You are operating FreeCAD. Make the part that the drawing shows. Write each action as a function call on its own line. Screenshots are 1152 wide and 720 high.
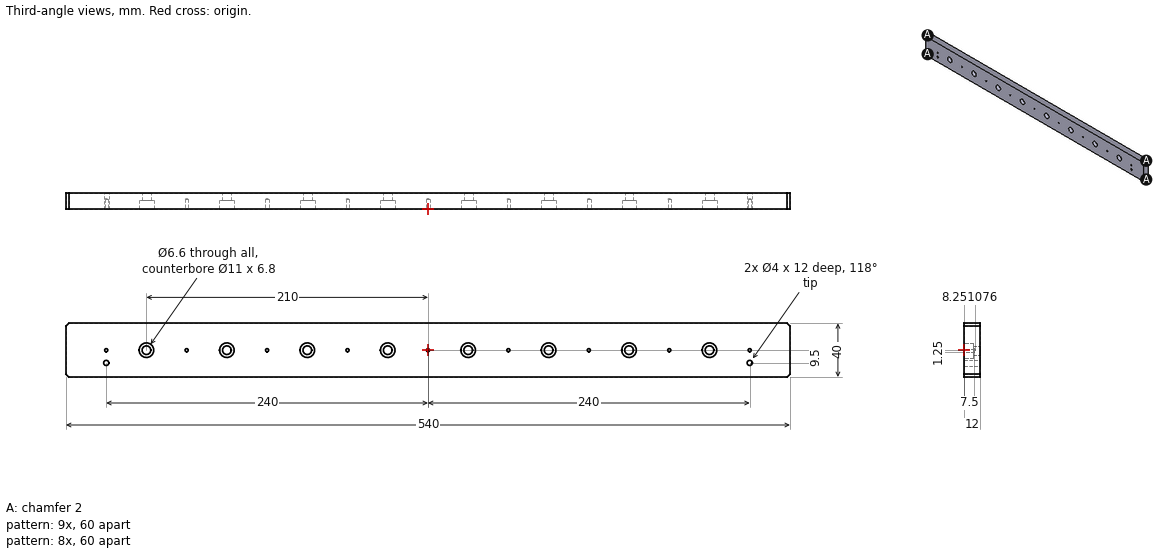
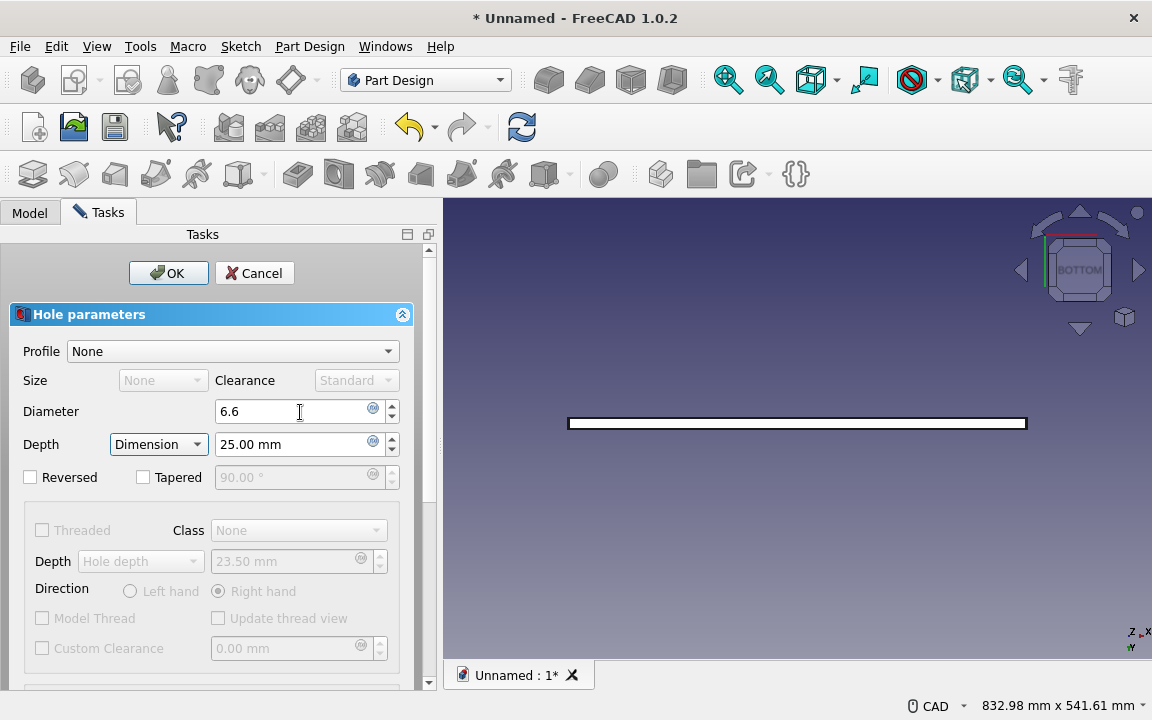
click(160, 444)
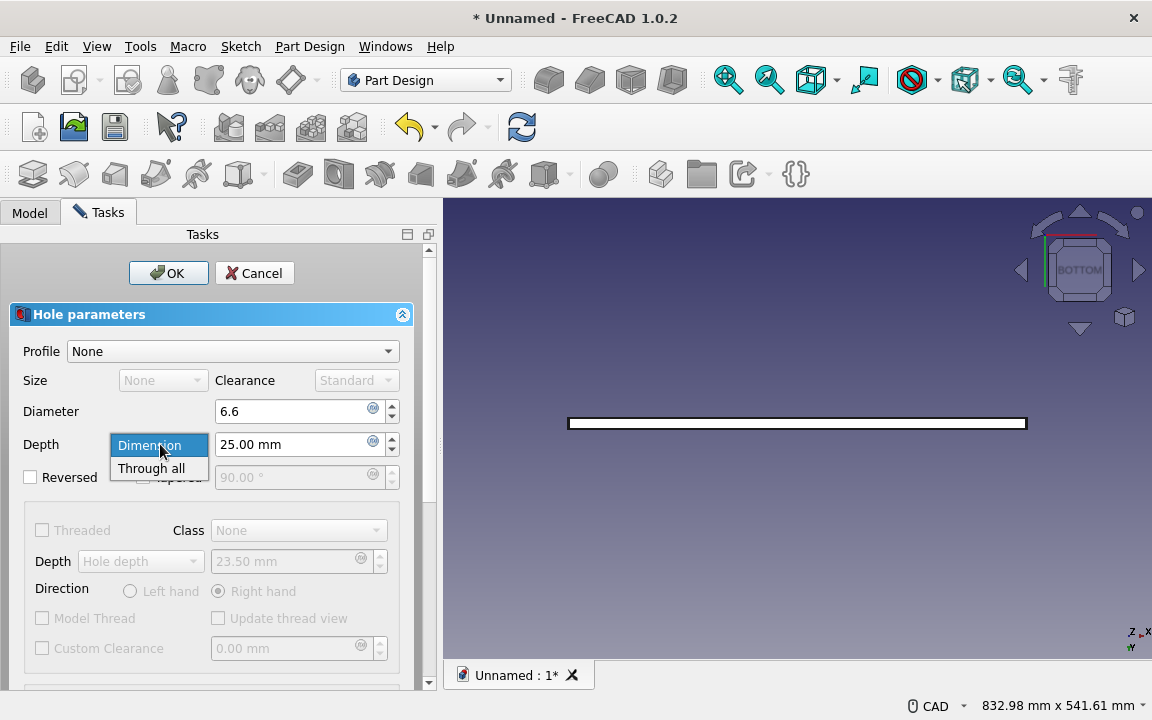
click(158, 468)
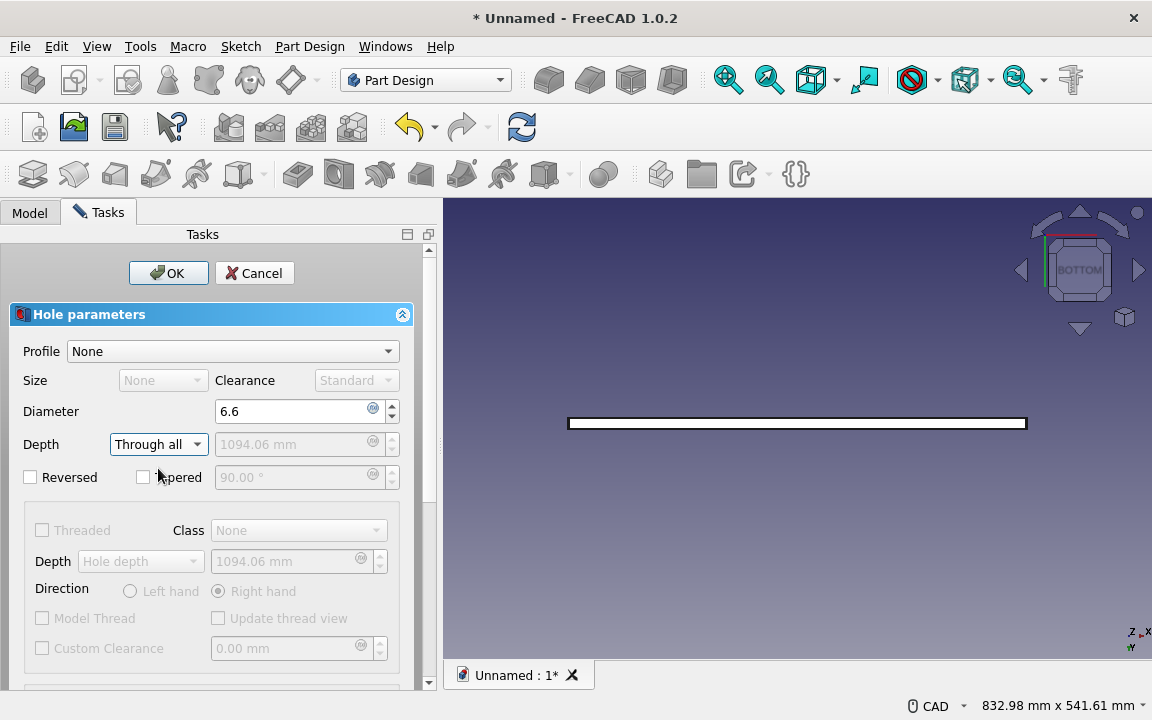
scroll(429, 467, down, 2)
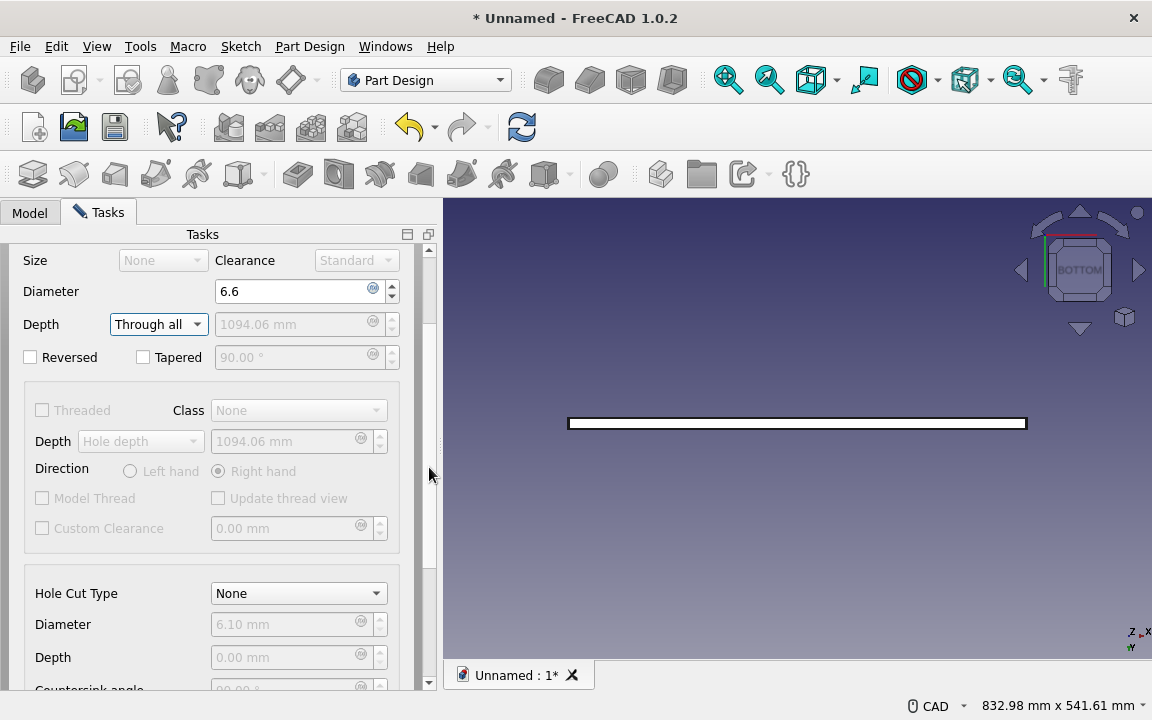
click(300, 594)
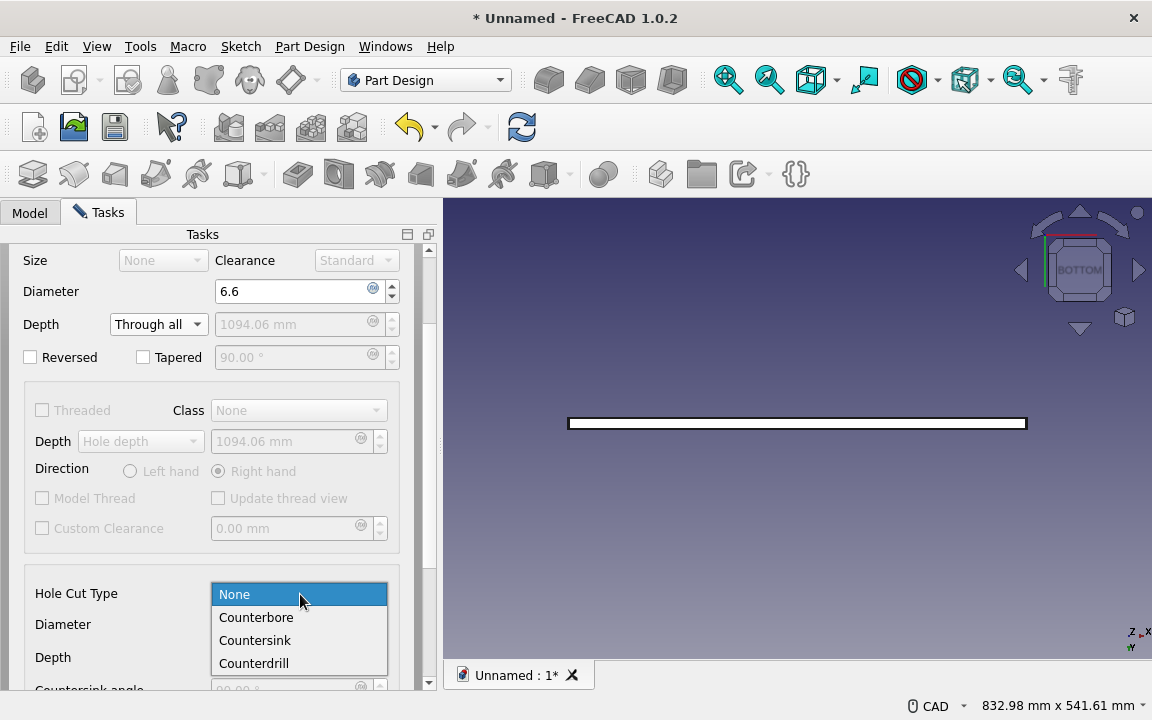
click(298, 618)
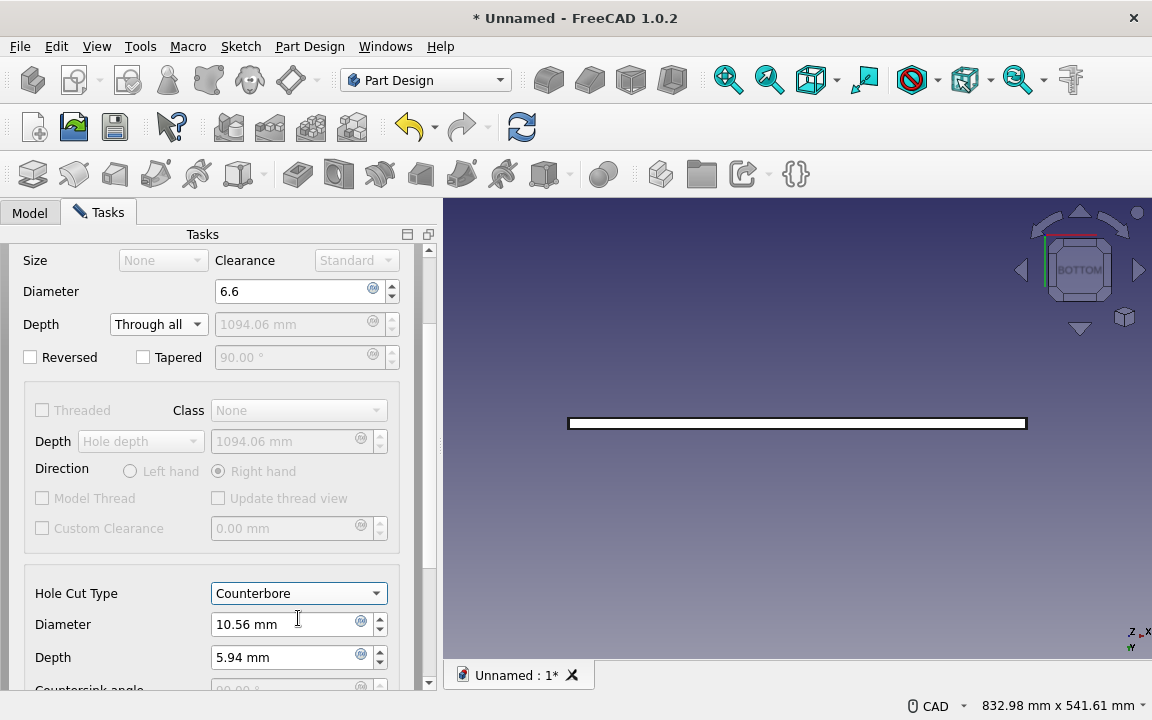
triple_click(292, 624)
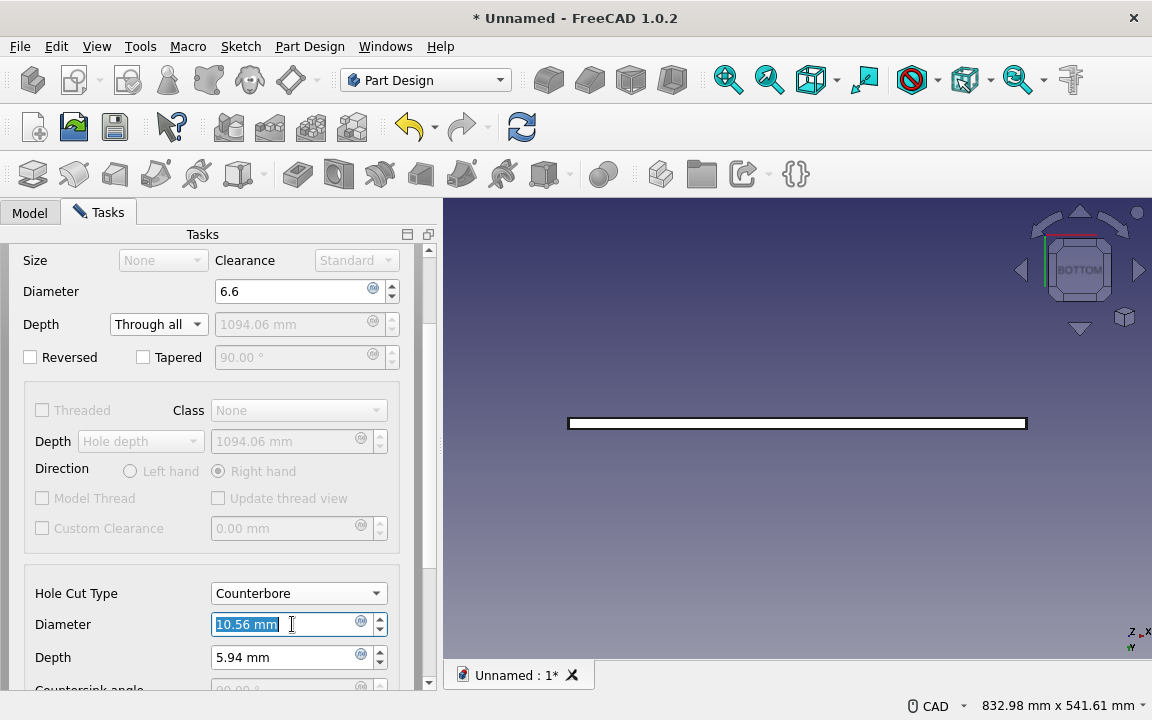
text(11)
key(Tab)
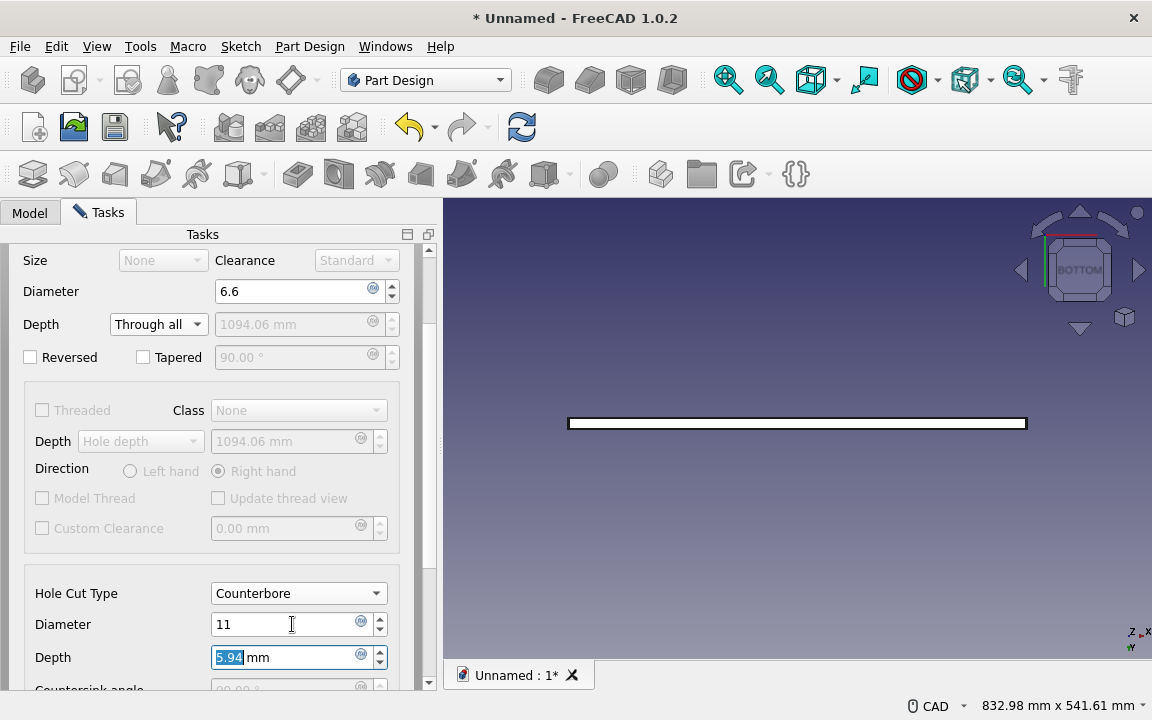
text(6.8)
key(Tab)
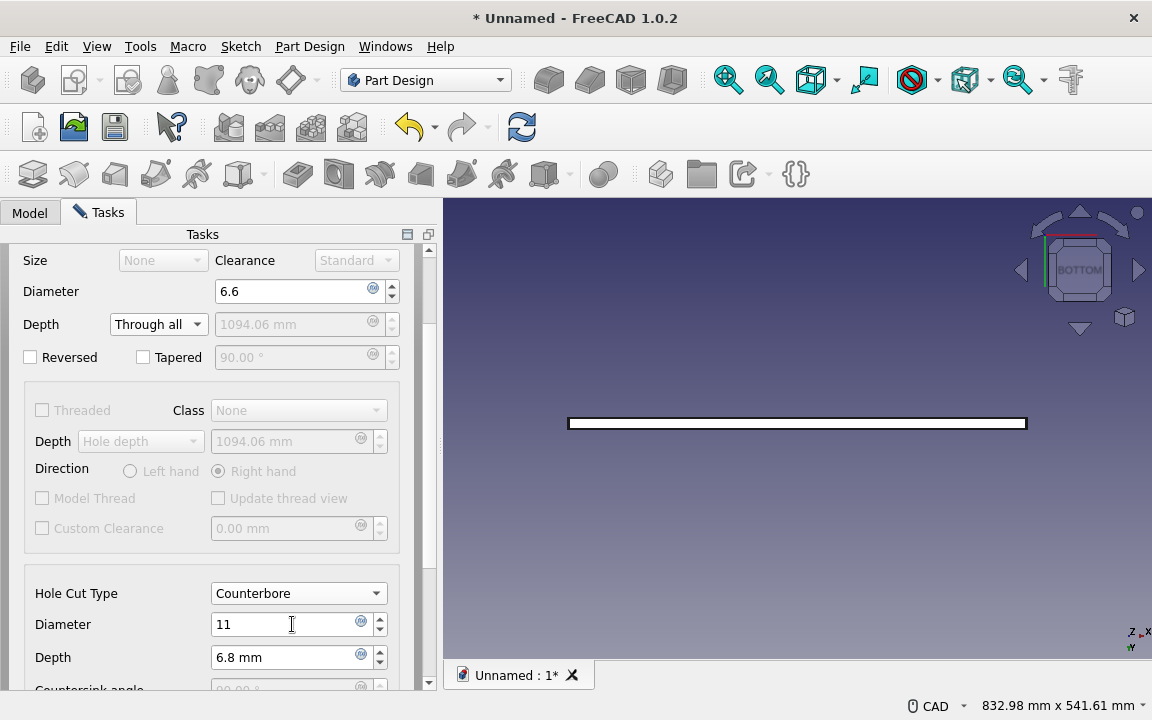
scroll(429, 467, up, 3)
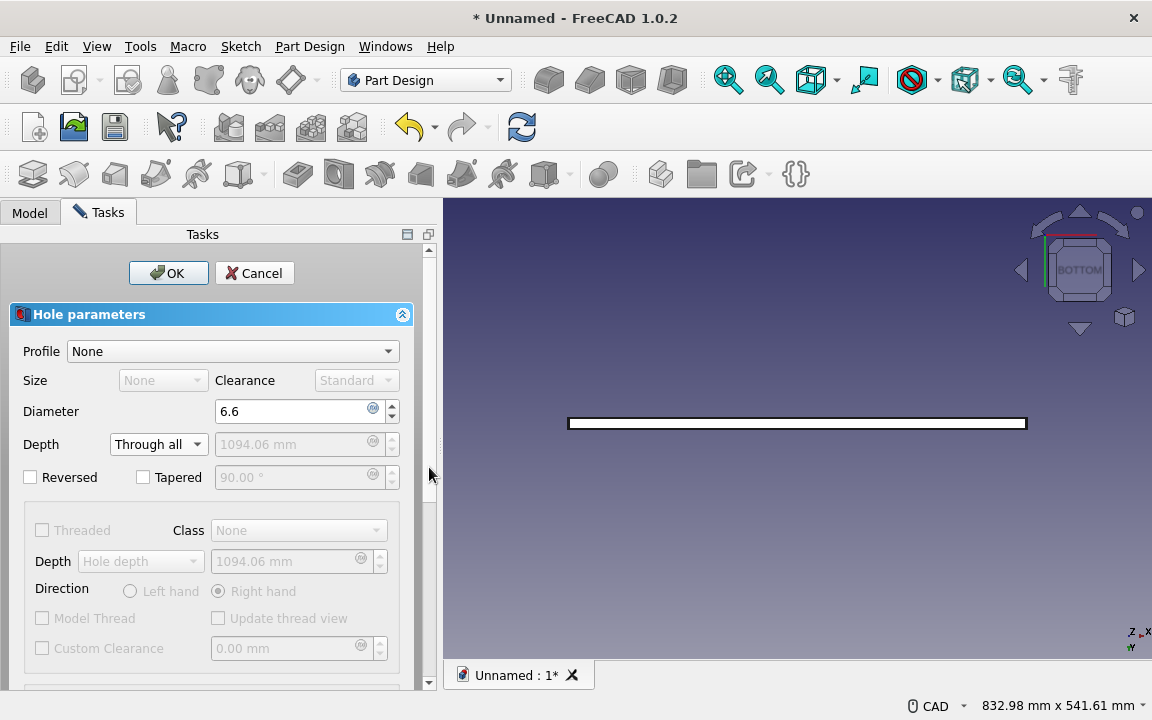
click(169, 273)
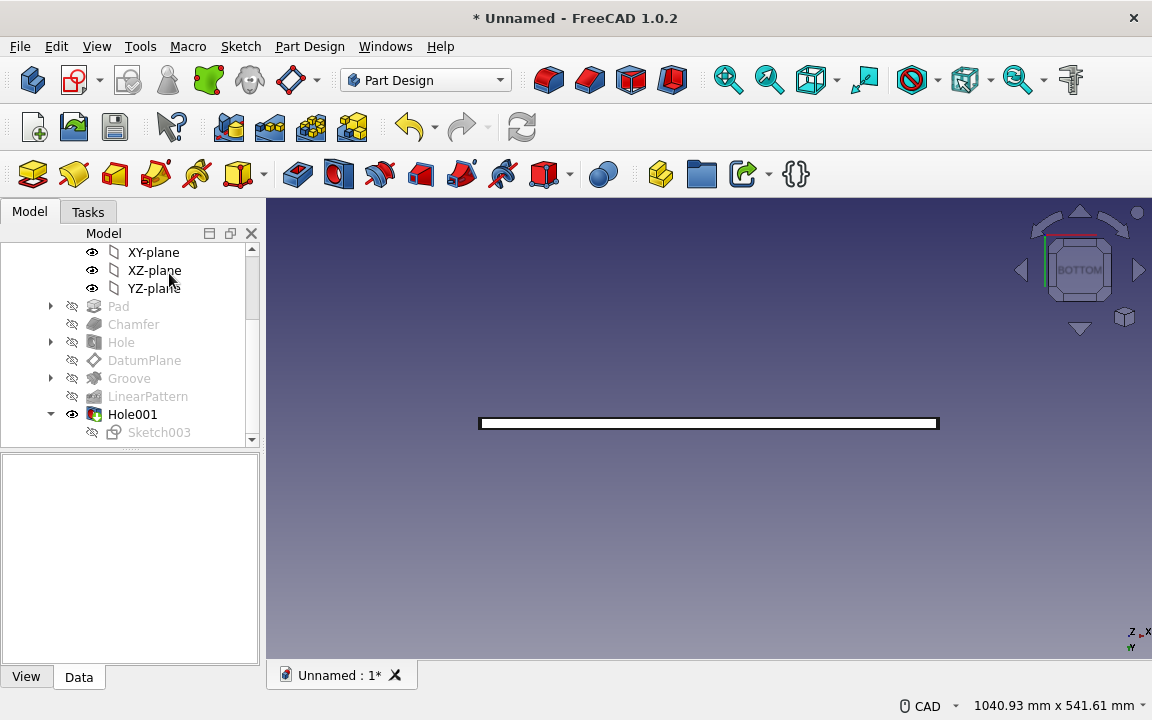
click(117, 414)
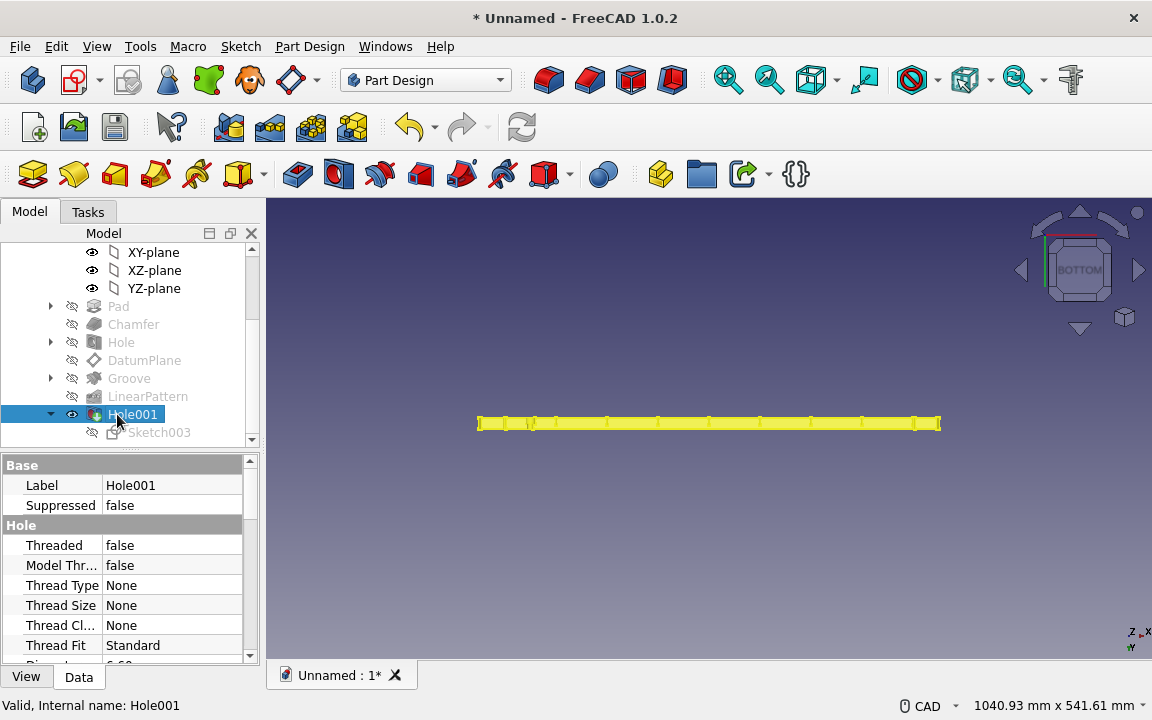
click(270, 128)